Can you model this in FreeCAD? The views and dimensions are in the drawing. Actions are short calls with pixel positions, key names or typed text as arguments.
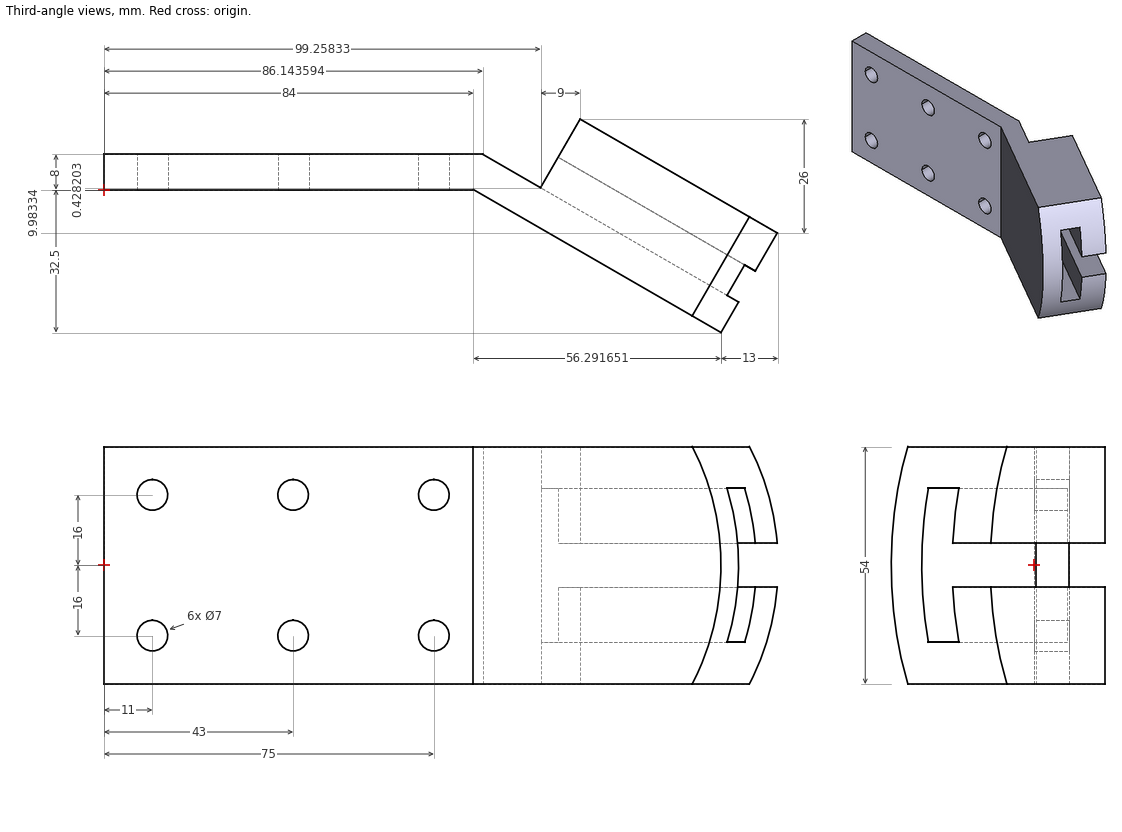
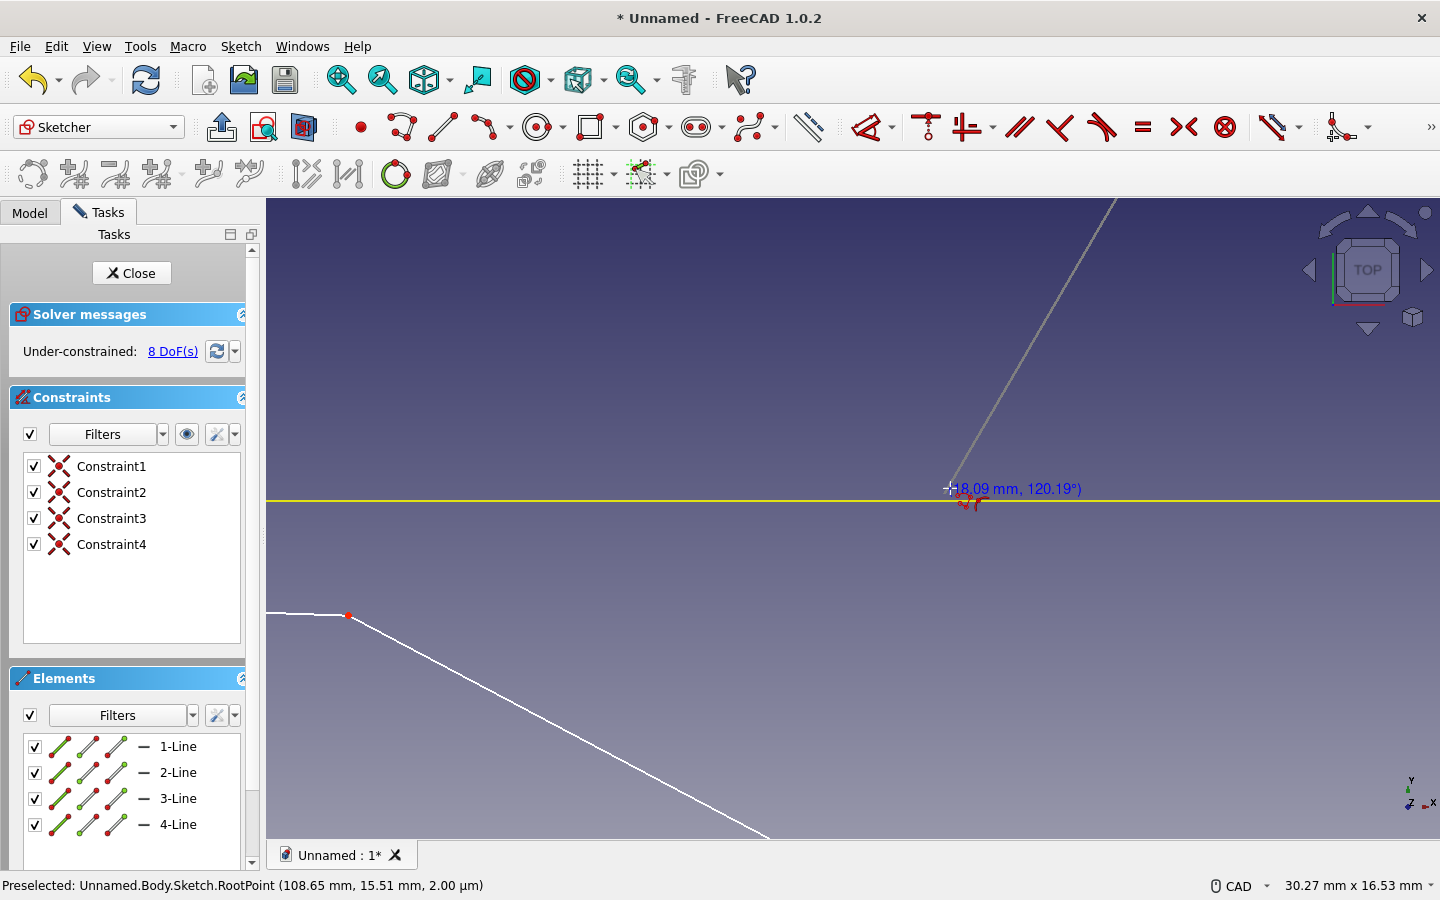
click(944, 484)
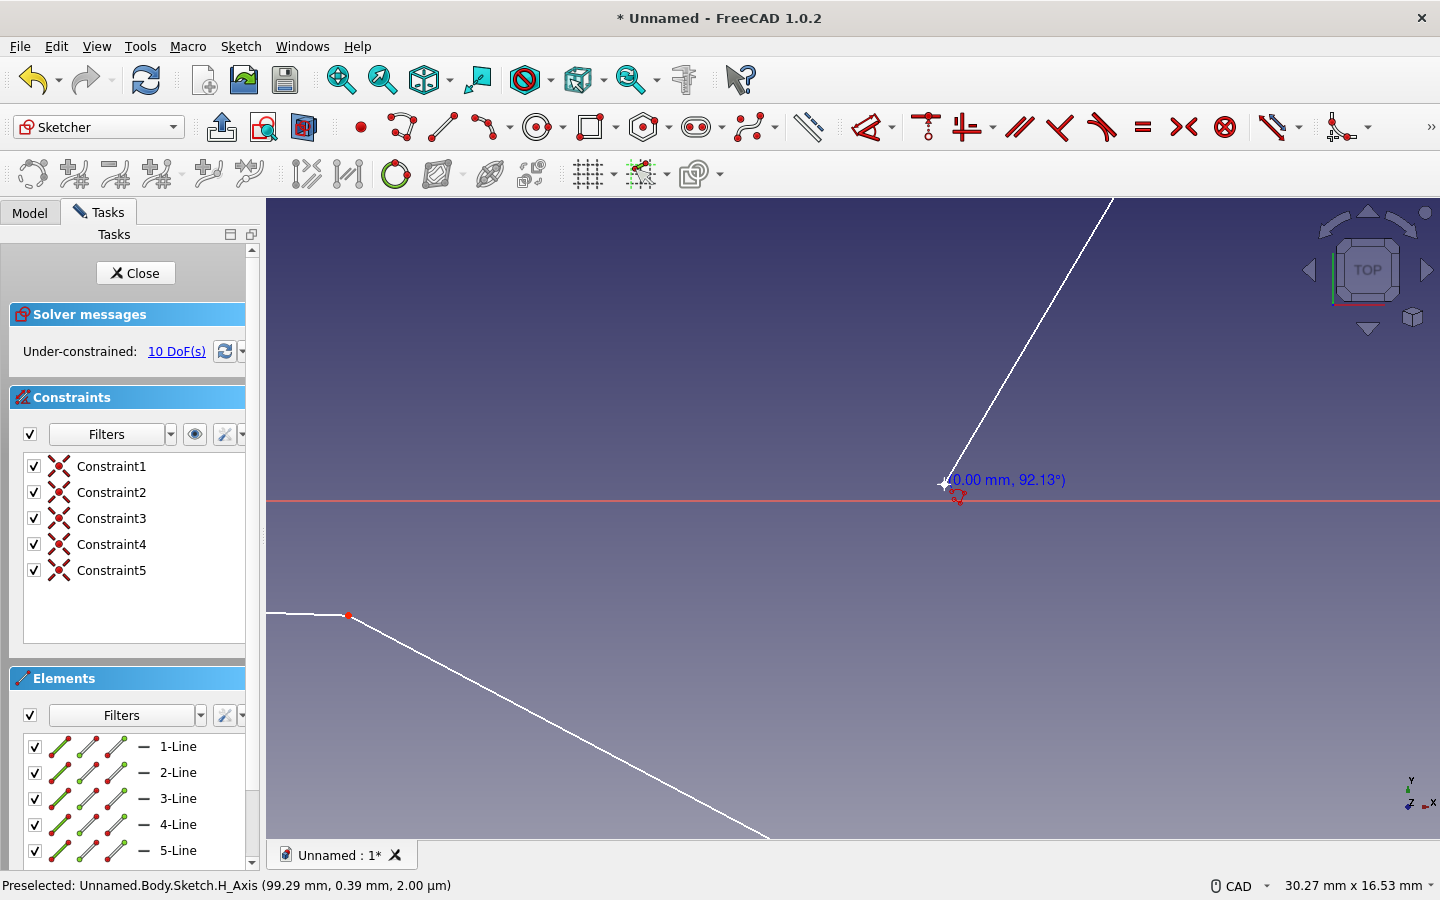
scroll(874, 481, down, 11)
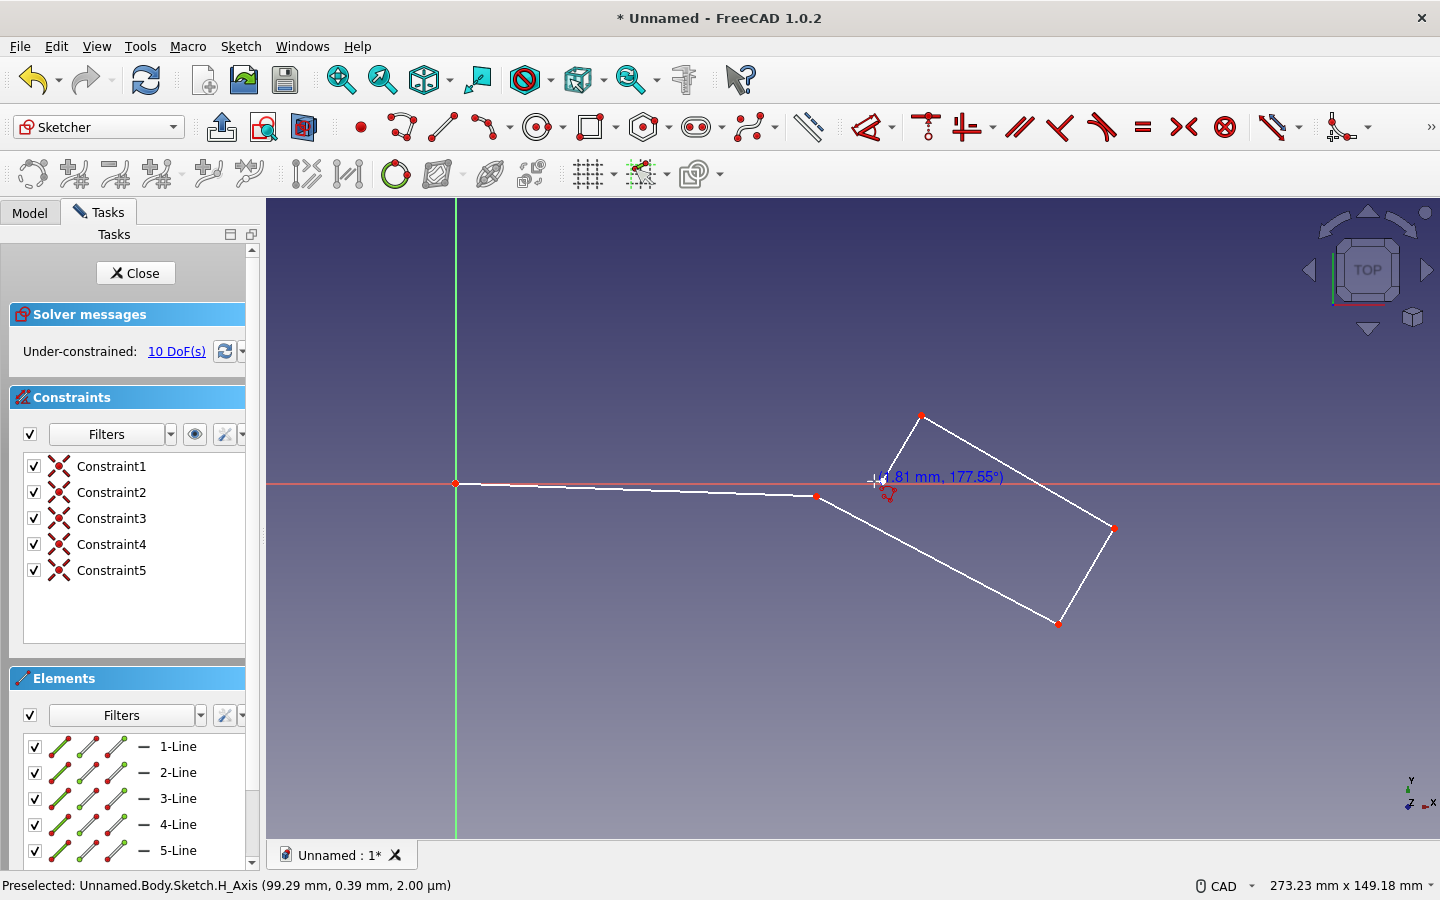
click(826, 449)
click(465, 449)
click(456, 484)
key(Escape)
key(Escape)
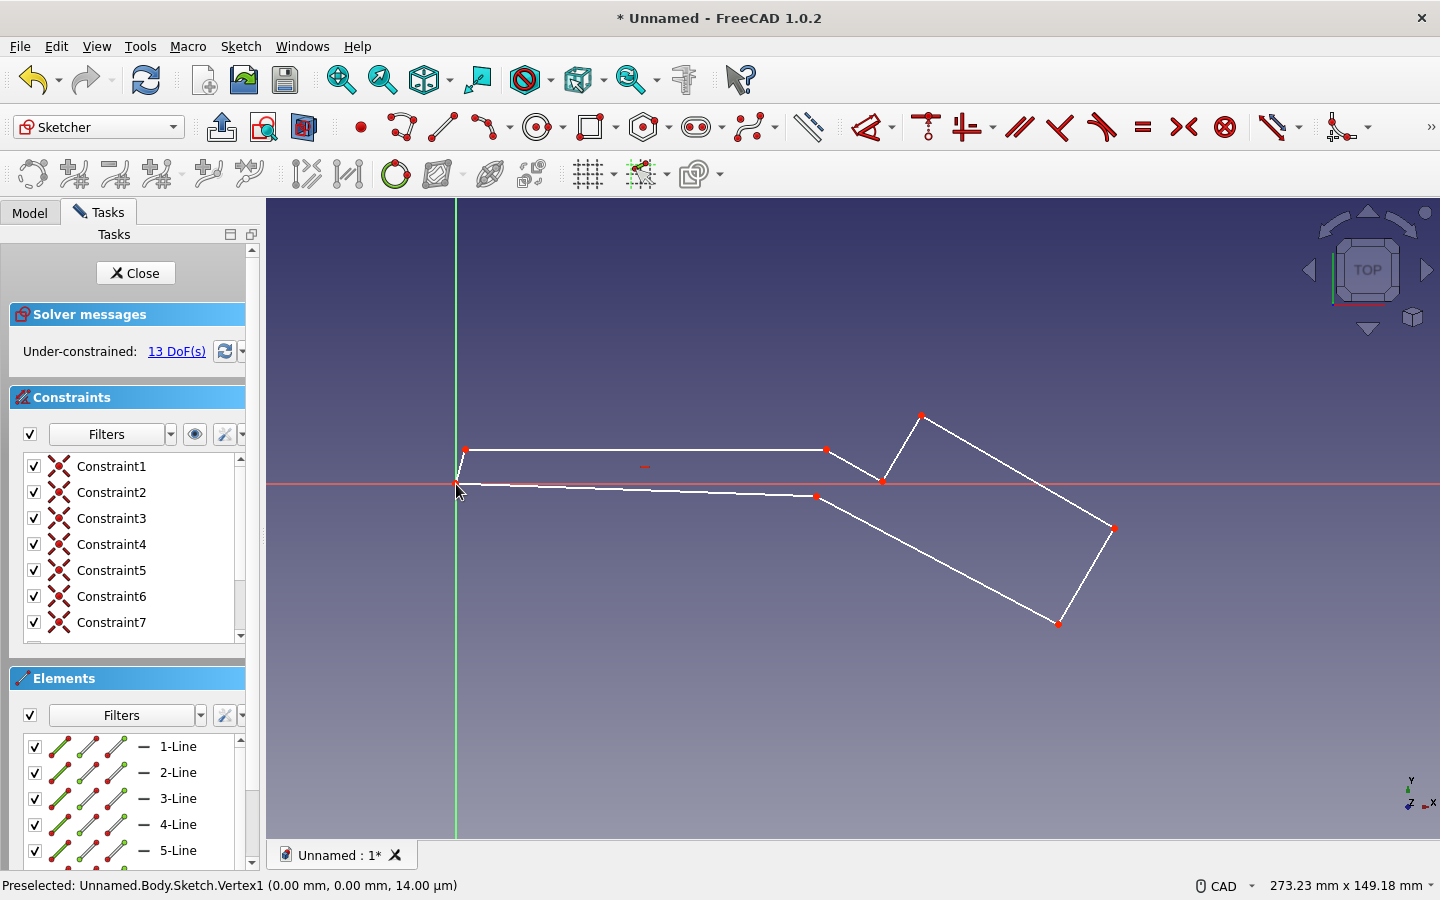
click(564, 487)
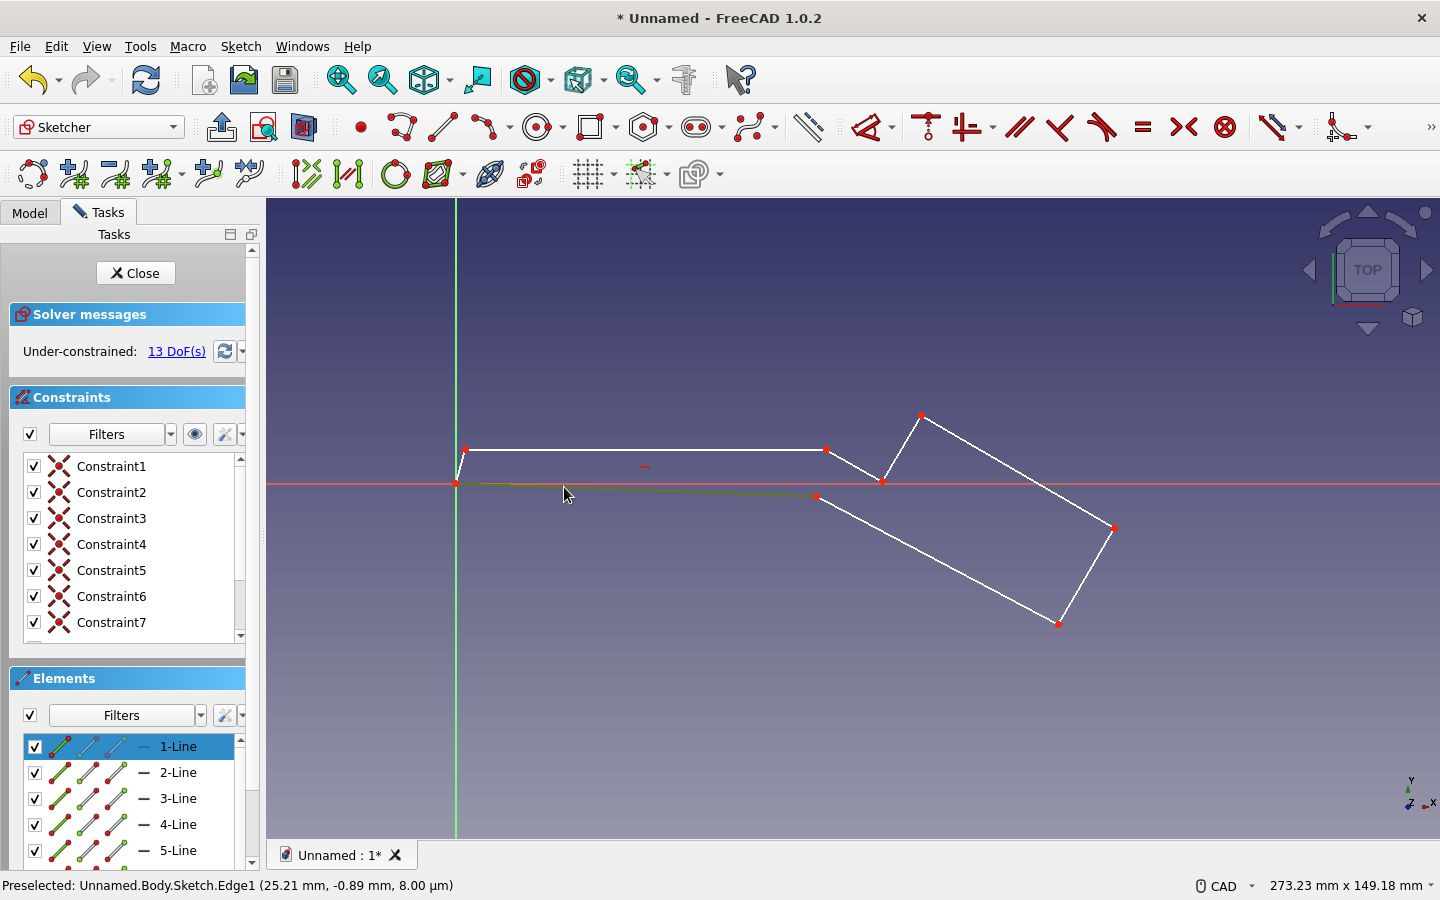
key(h)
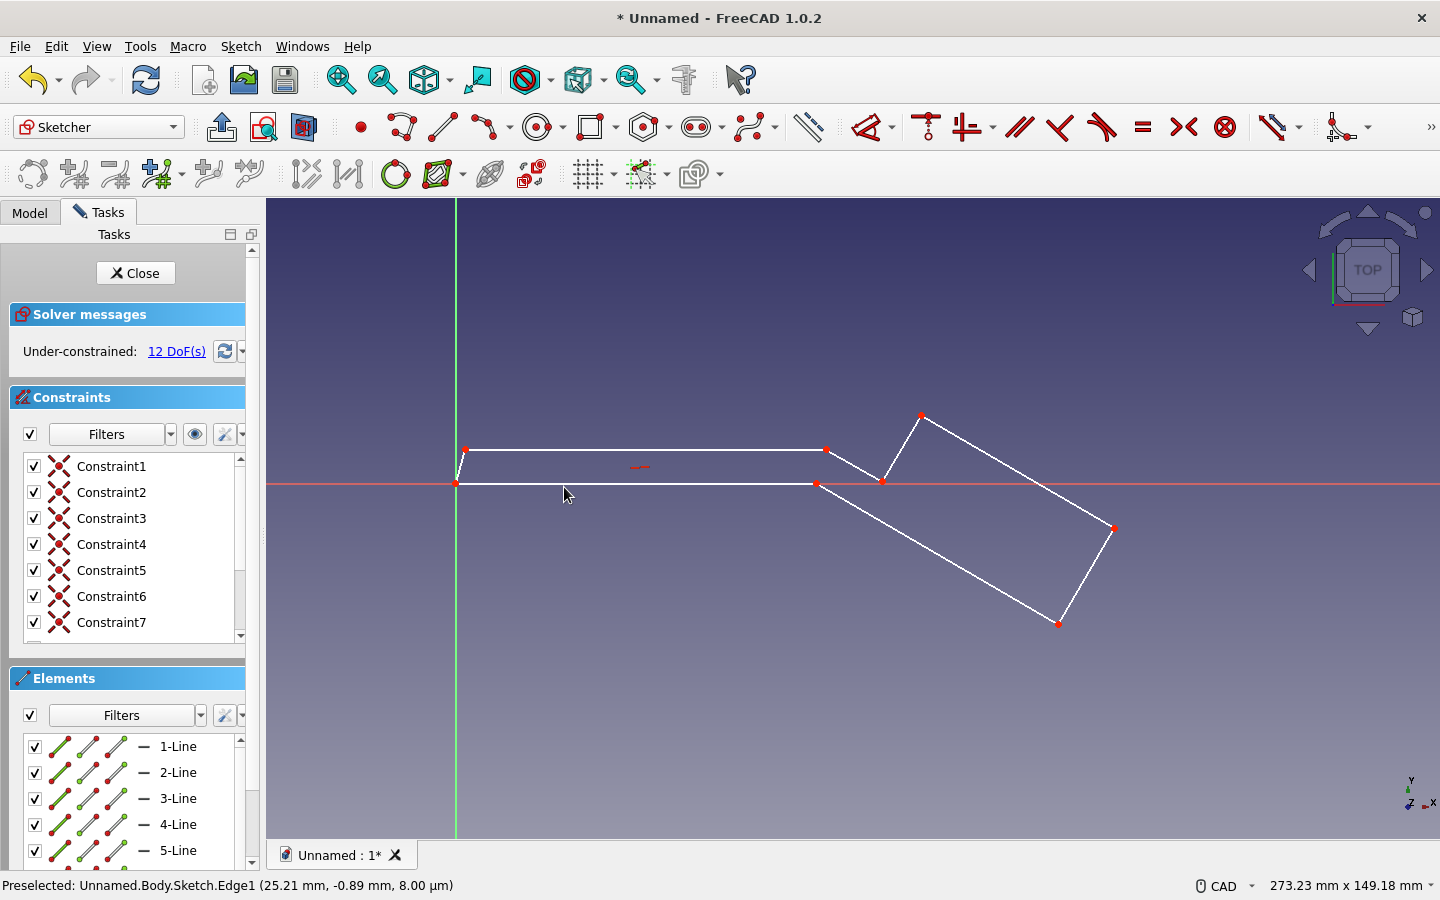
scroll(459, 474, up, 2)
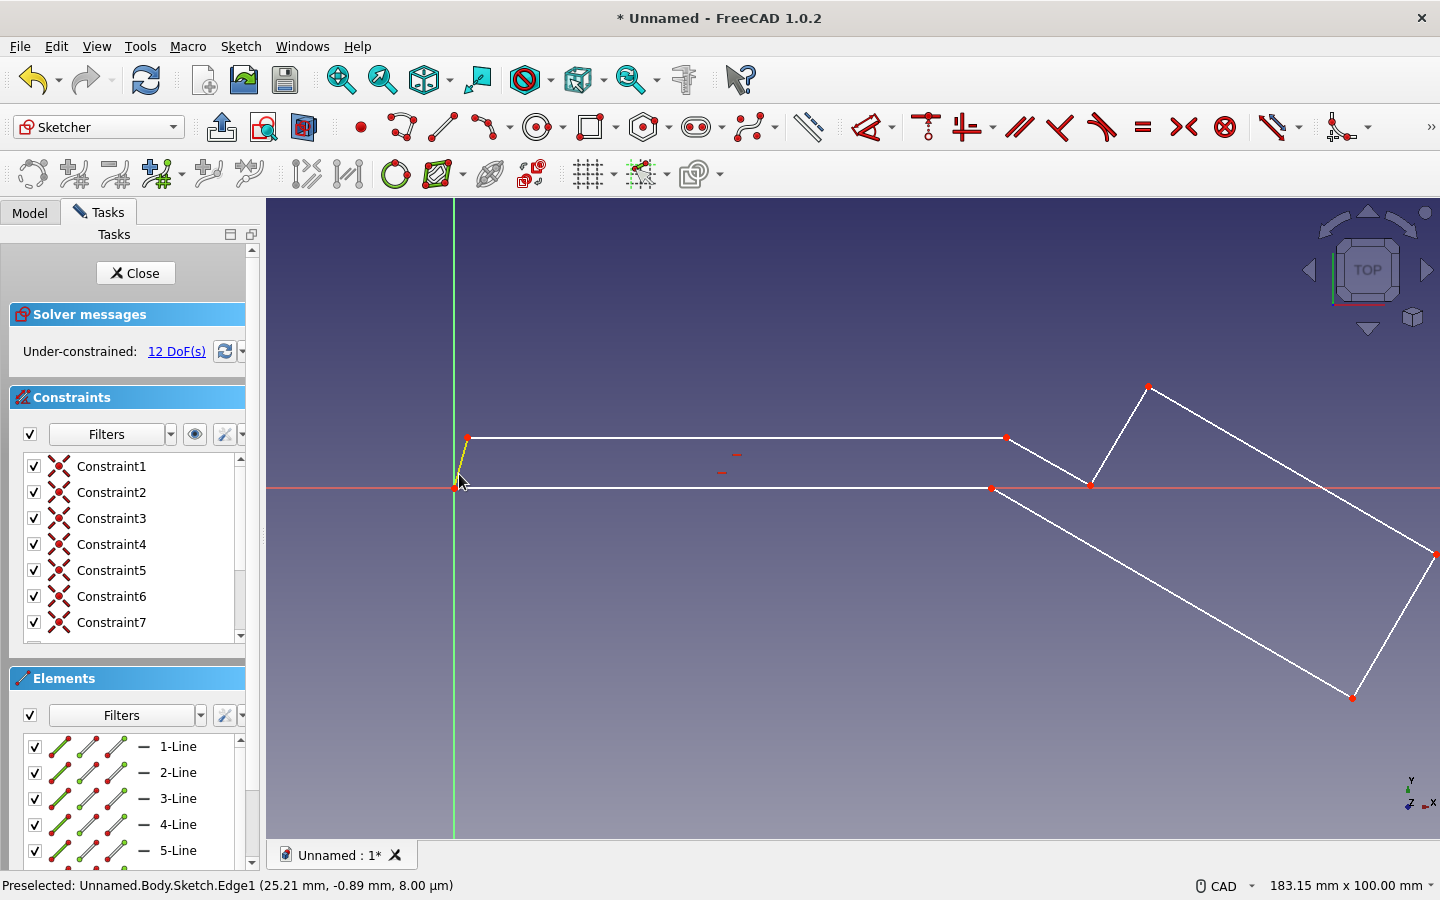
click(458, 473)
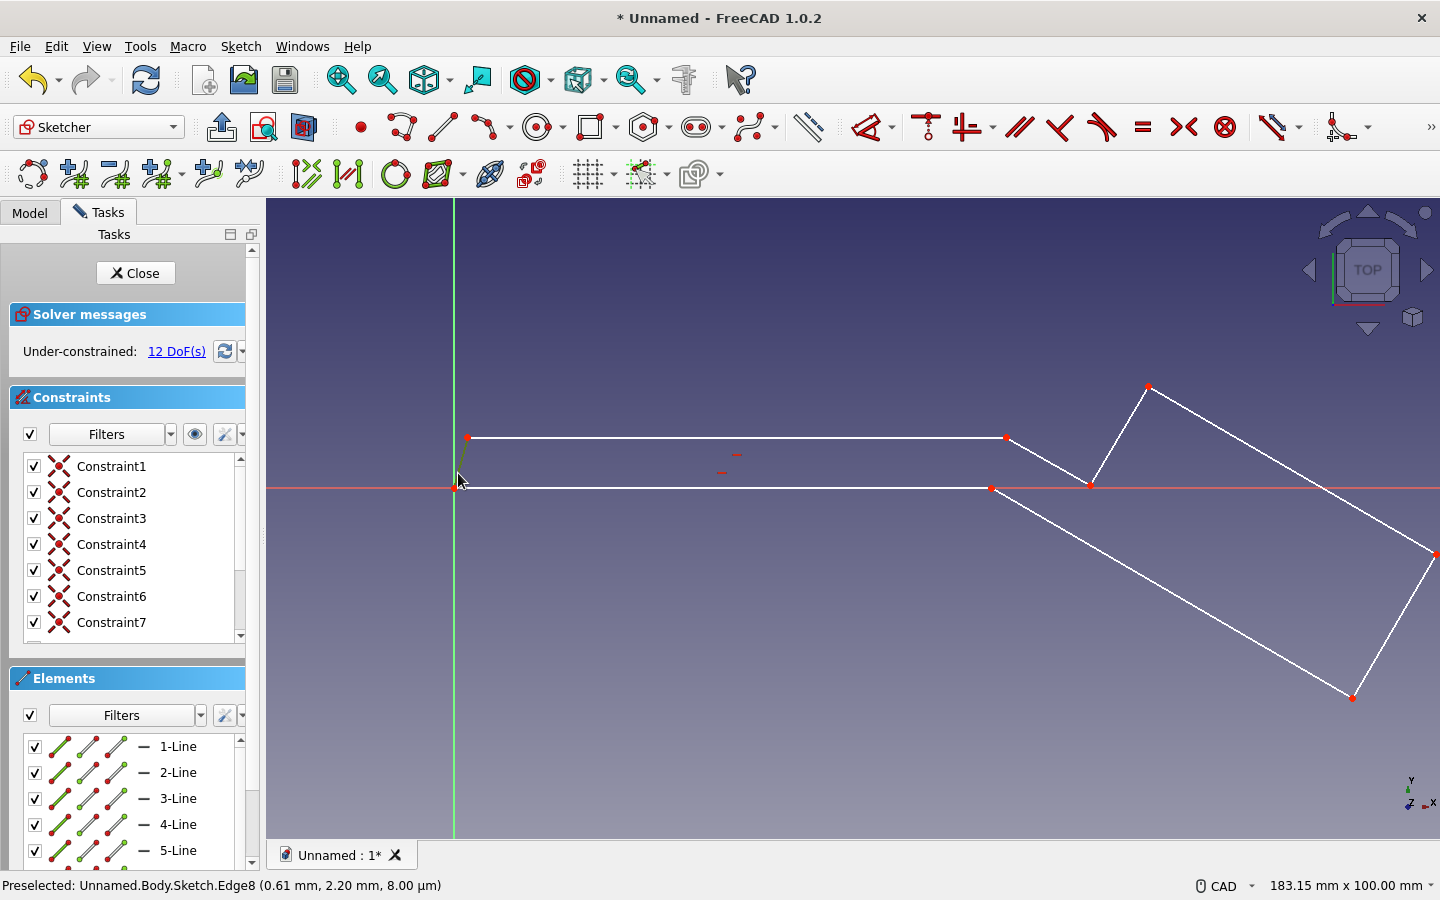
key(v)